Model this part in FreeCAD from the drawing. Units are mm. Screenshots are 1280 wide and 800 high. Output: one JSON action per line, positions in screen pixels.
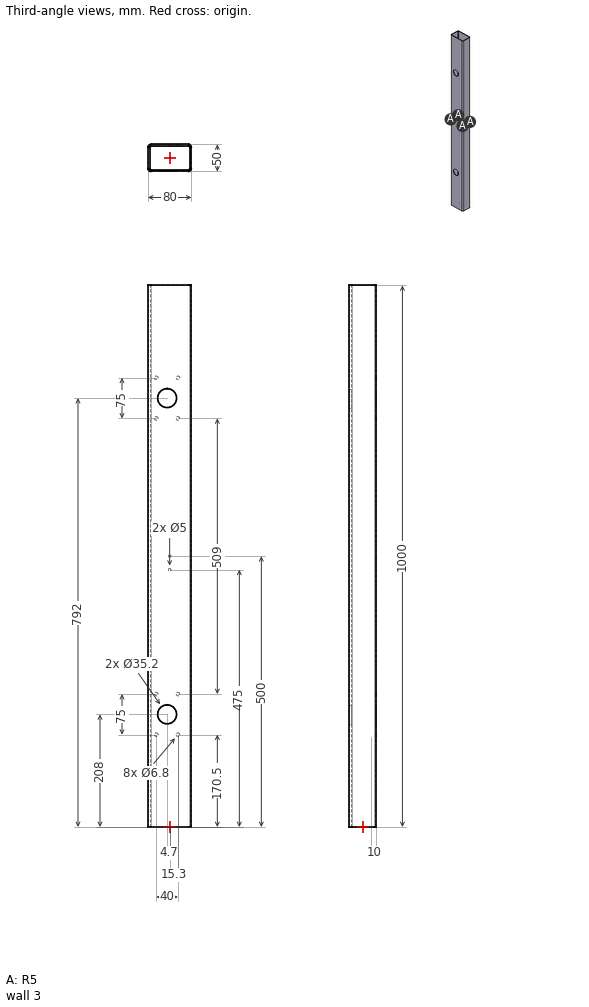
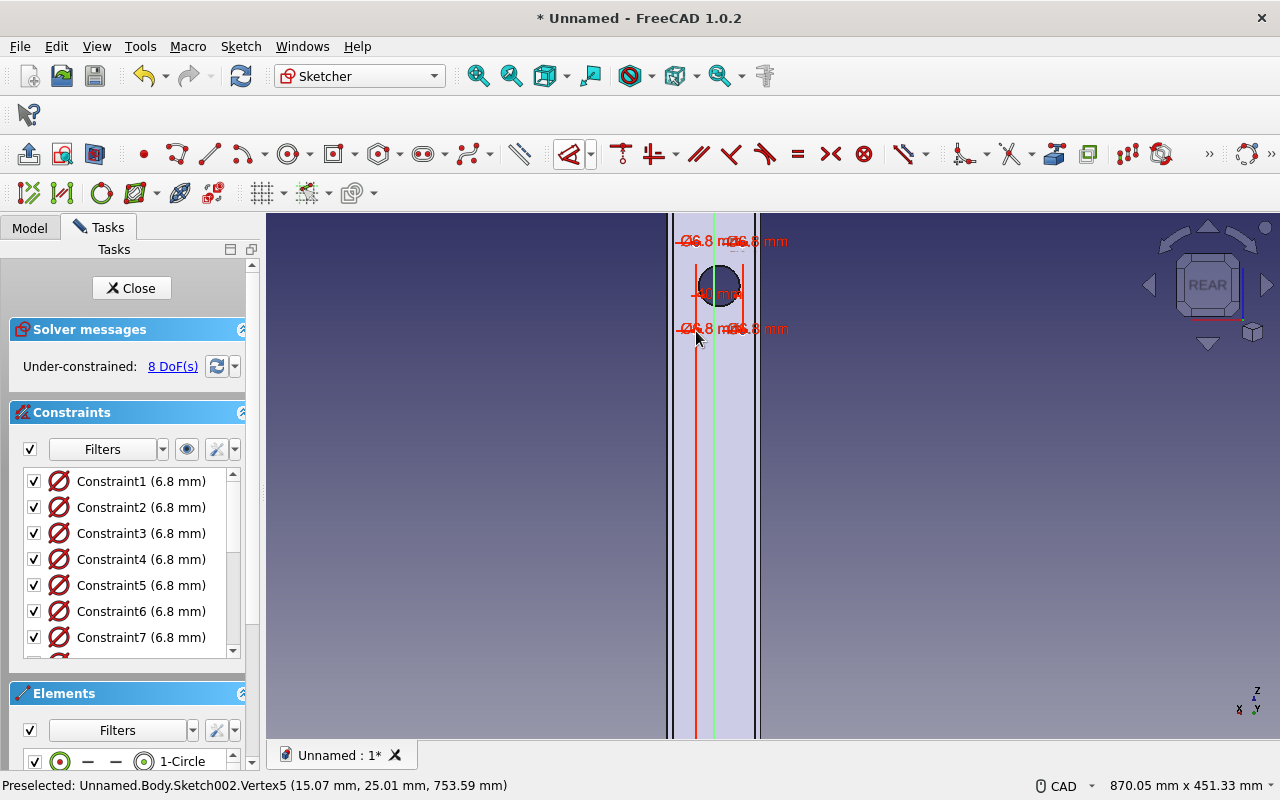
{"action": "left_click", "coordinate": [742, 244]}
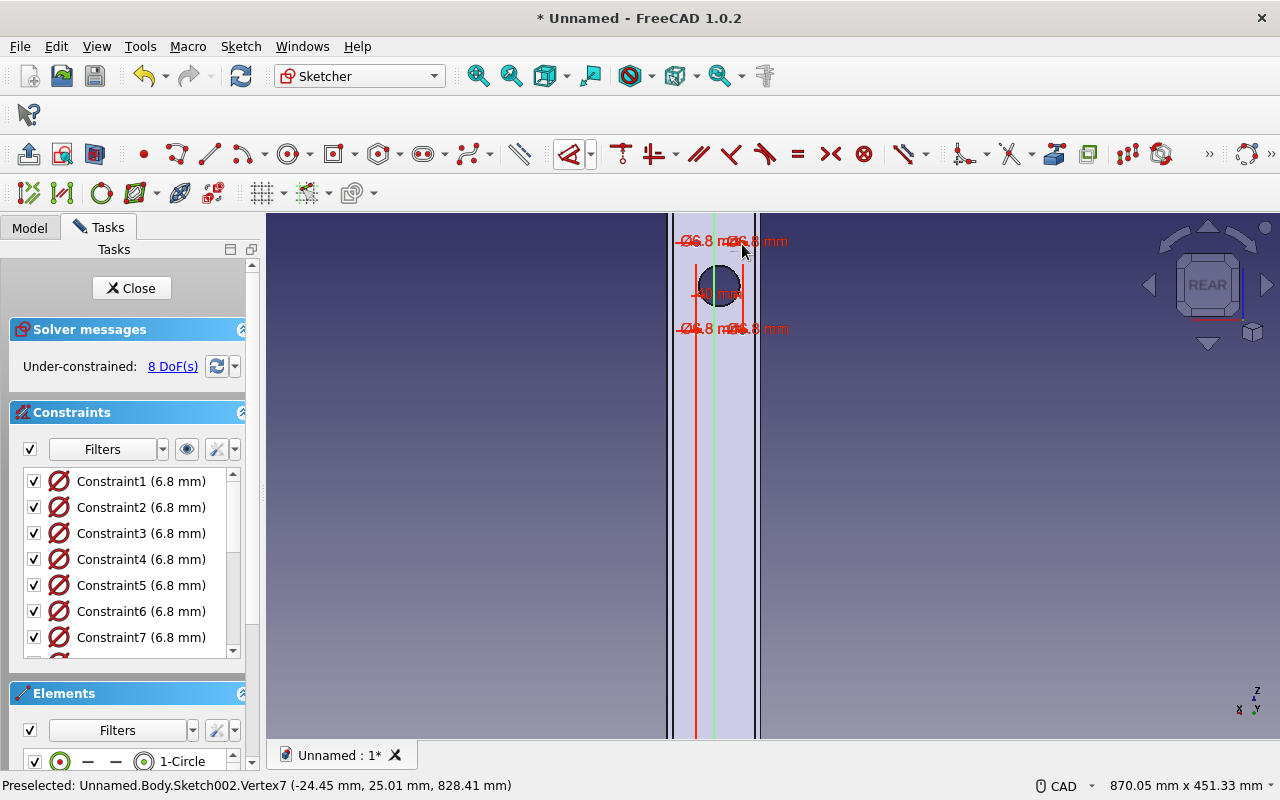
{"action": "key", "text": "l"}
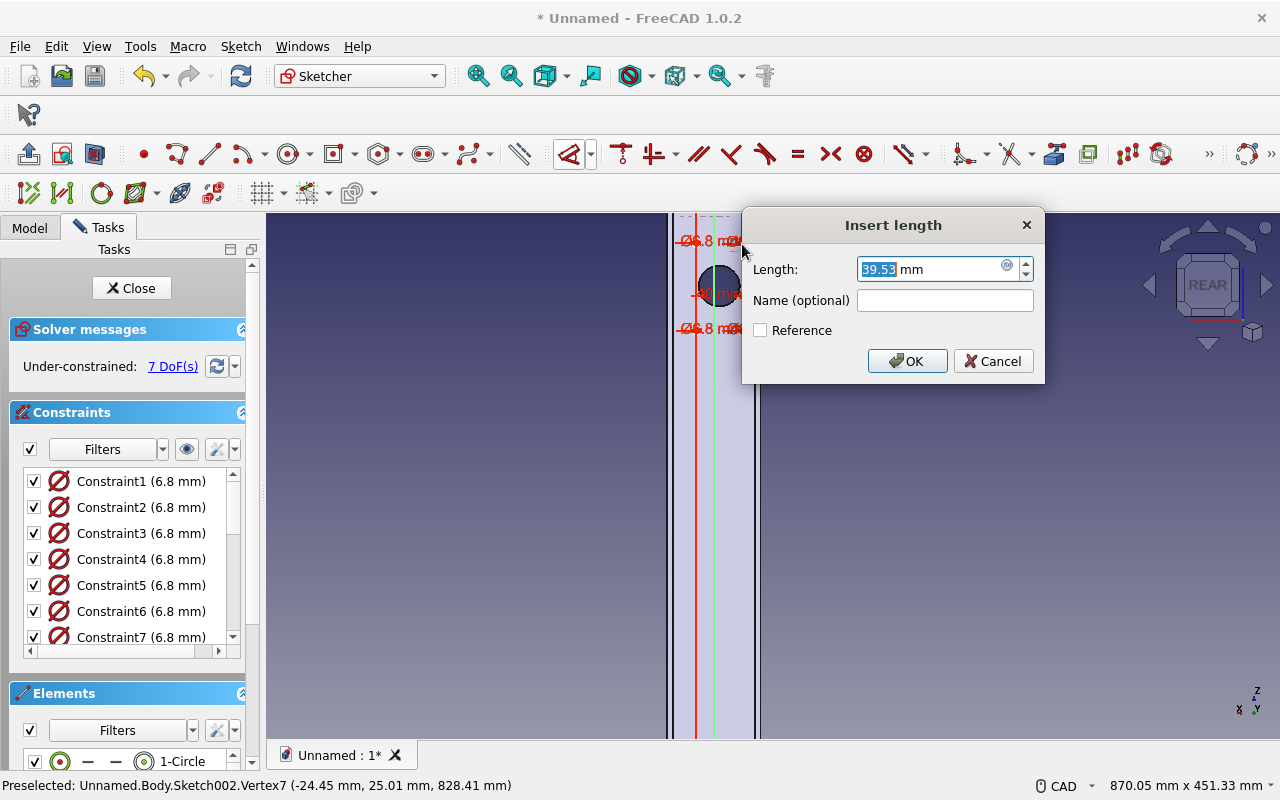
{"action": "type", "text": "40"}
{"action": "key", "text": "Return"}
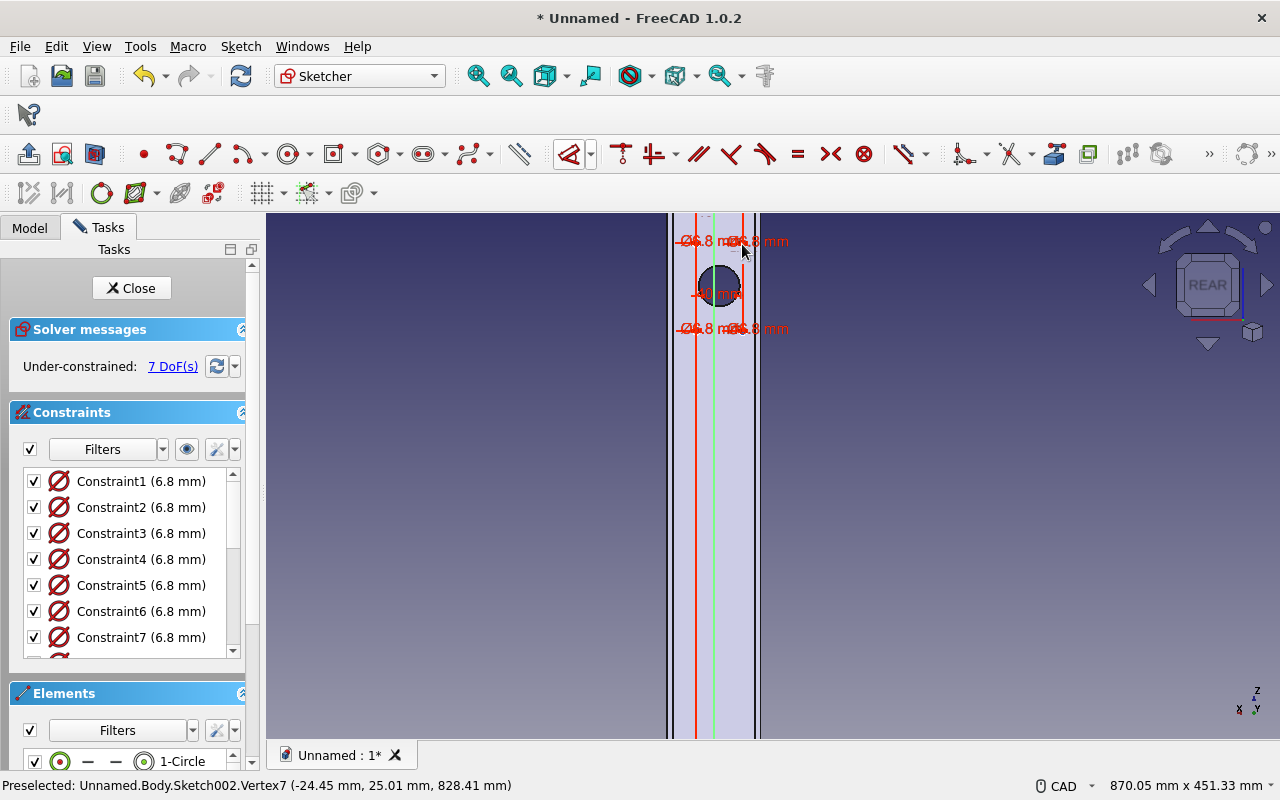
{"action": "left_click", "coordinate": [743, 331]}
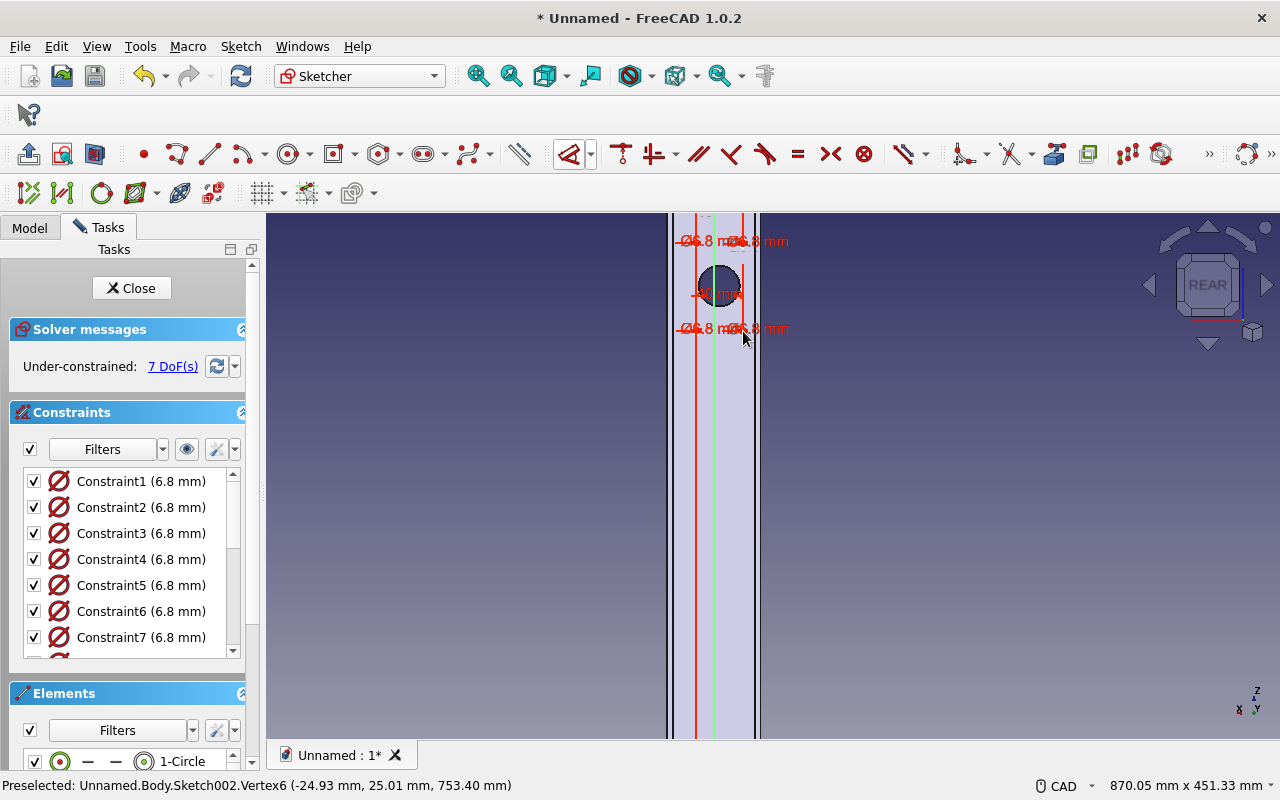
{"action": "left_click", "coordinate": [743, 244]}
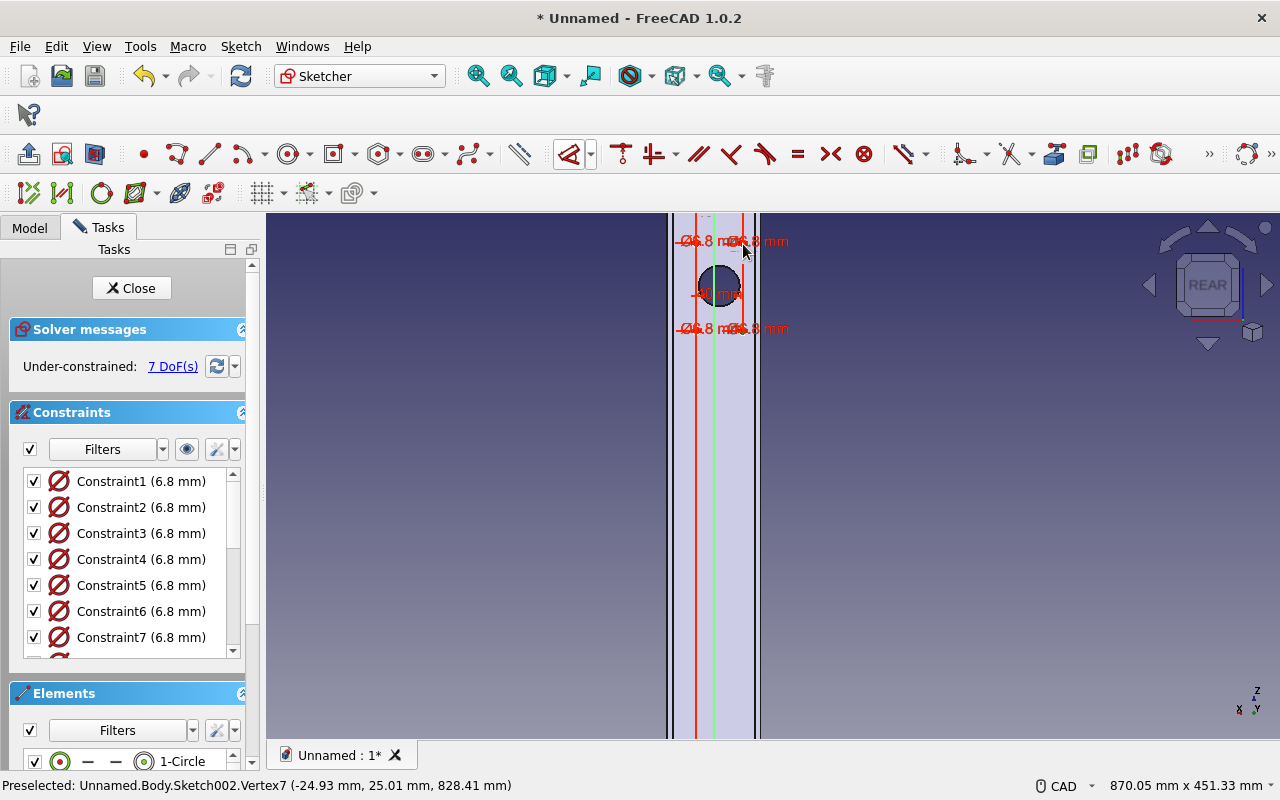
{"action": "key", "text": "i"}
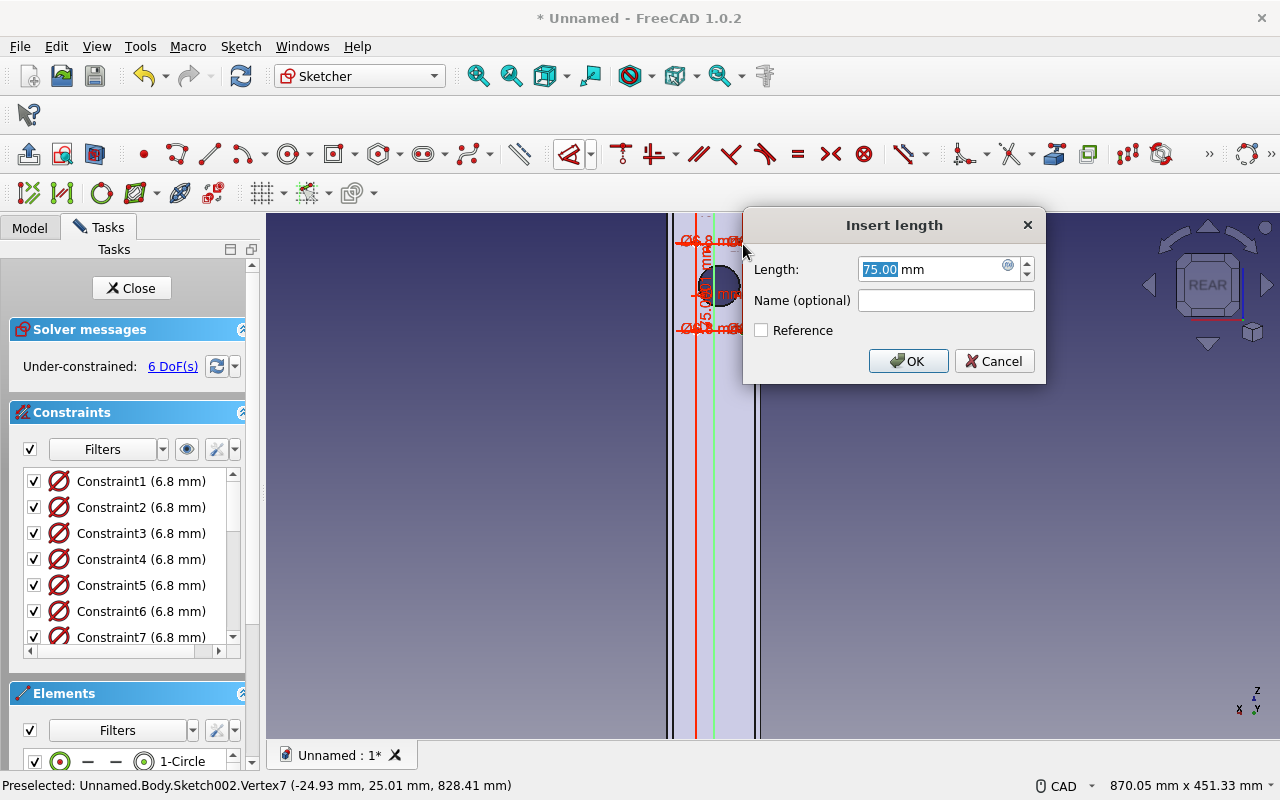
{"action": "type", "text": "75"}
{"action": "key", "text": "Return"}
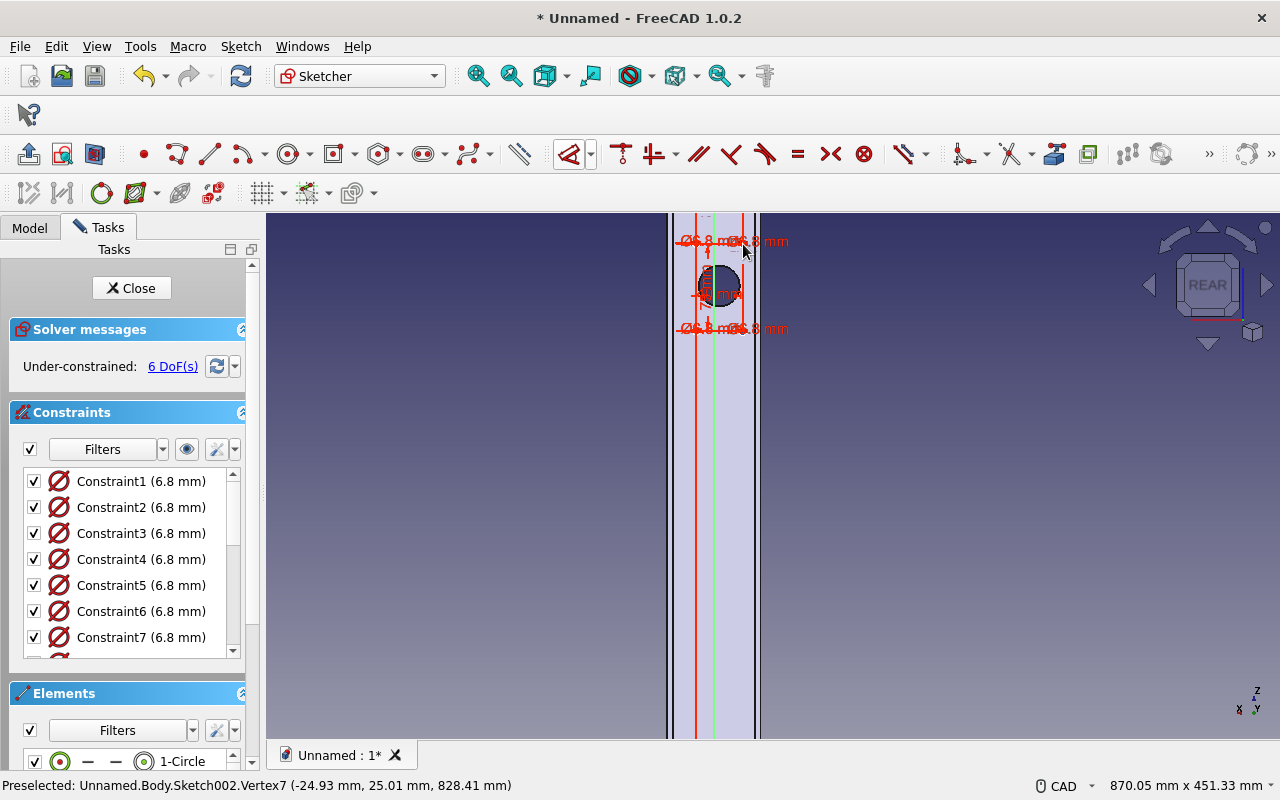
{"action": "left_click", "coordinate": [696, 331]}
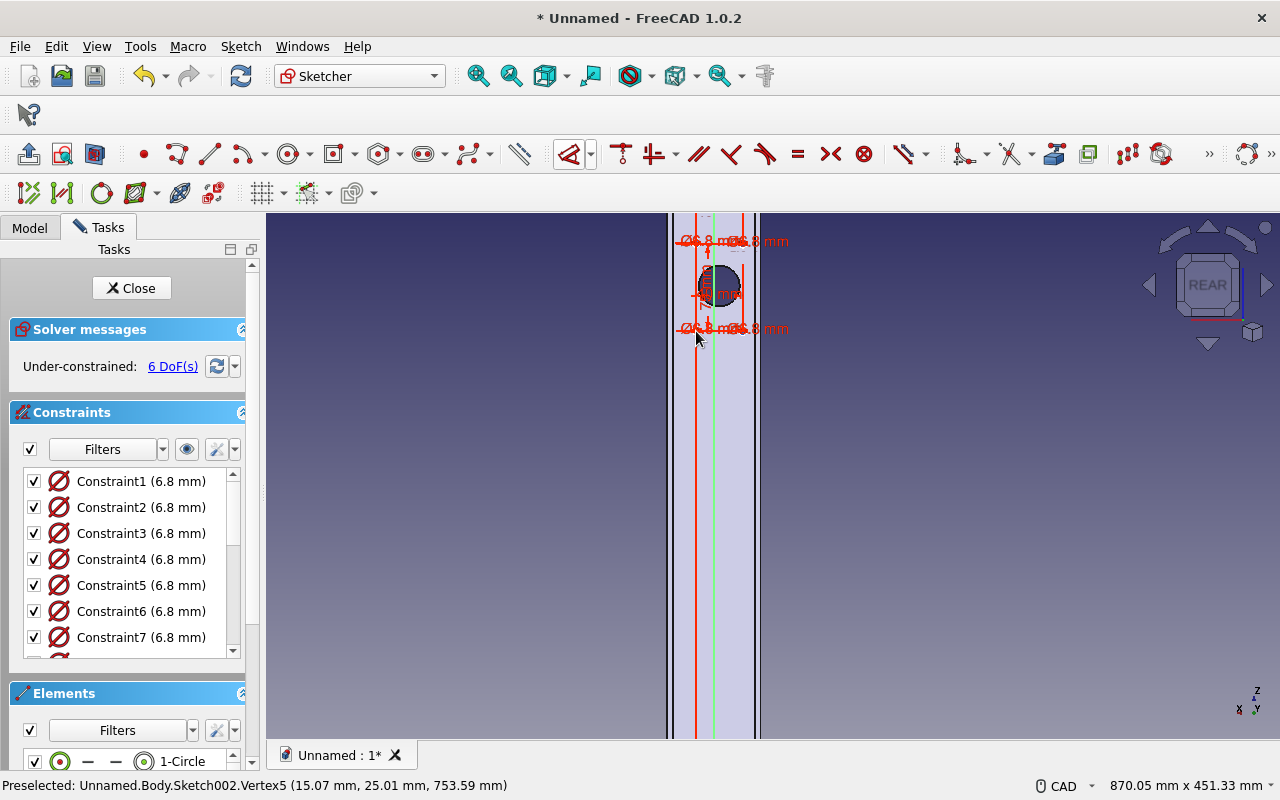
{"action": "left_click", "coordinate": [743, 244]}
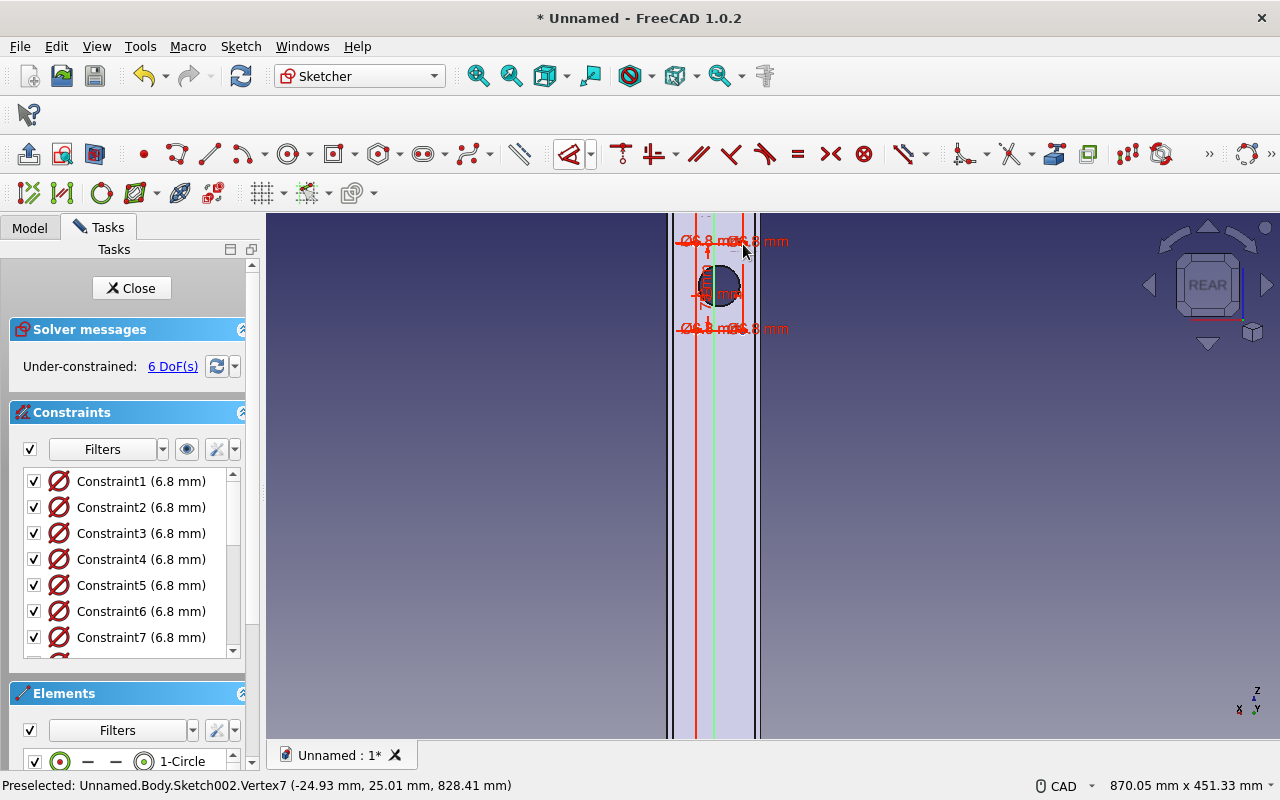
{"action": "left_click", "coordinate": [590, 154]}